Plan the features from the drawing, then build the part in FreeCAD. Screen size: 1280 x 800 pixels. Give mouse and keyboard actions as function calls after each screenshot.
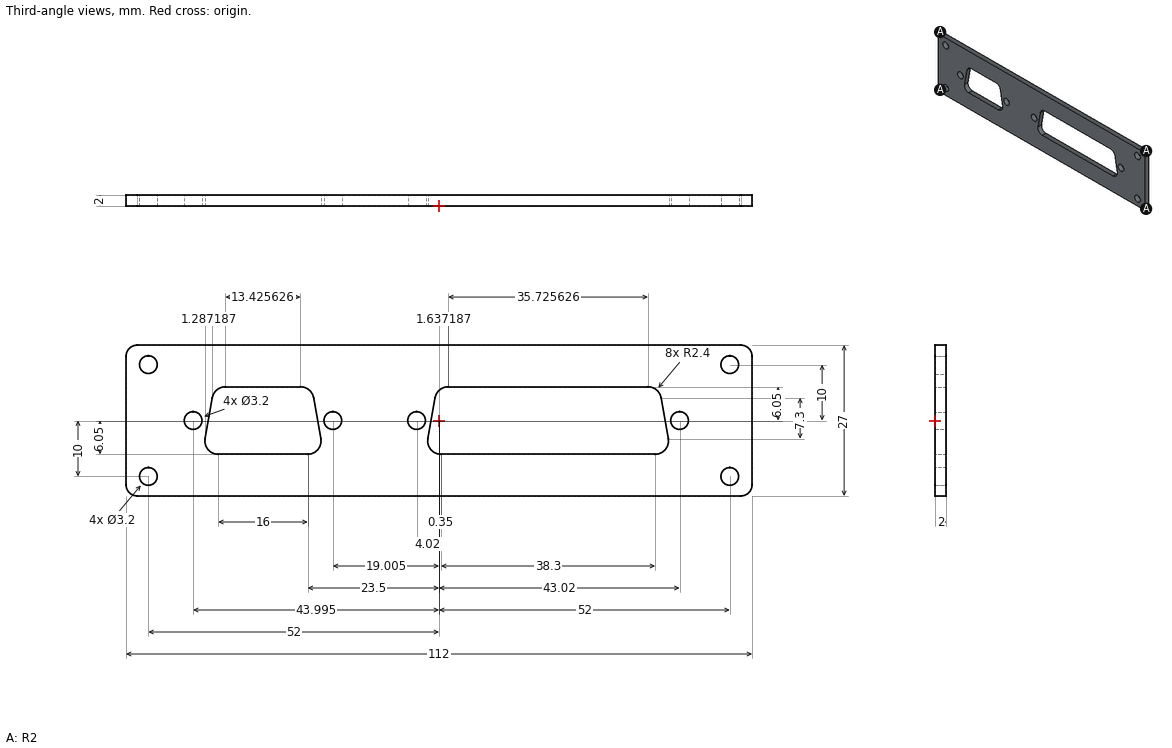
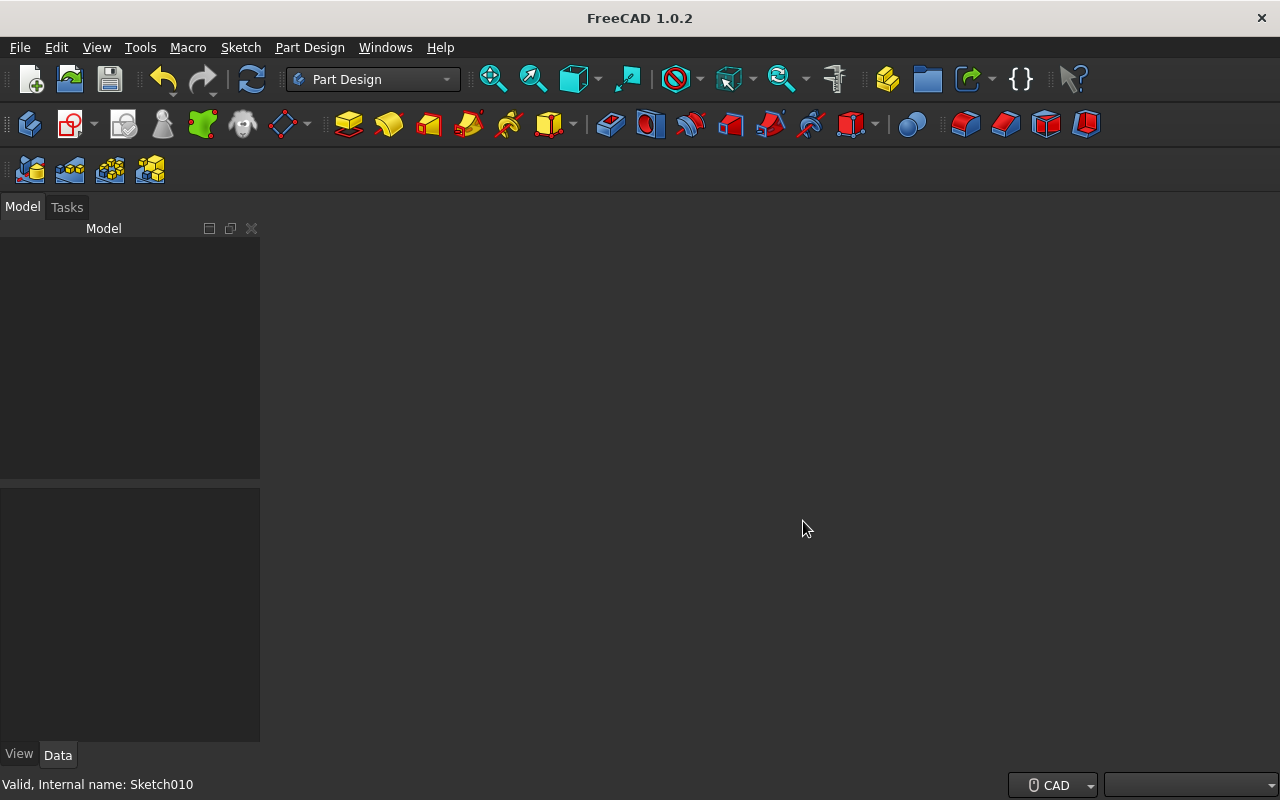
key(ctrl+n)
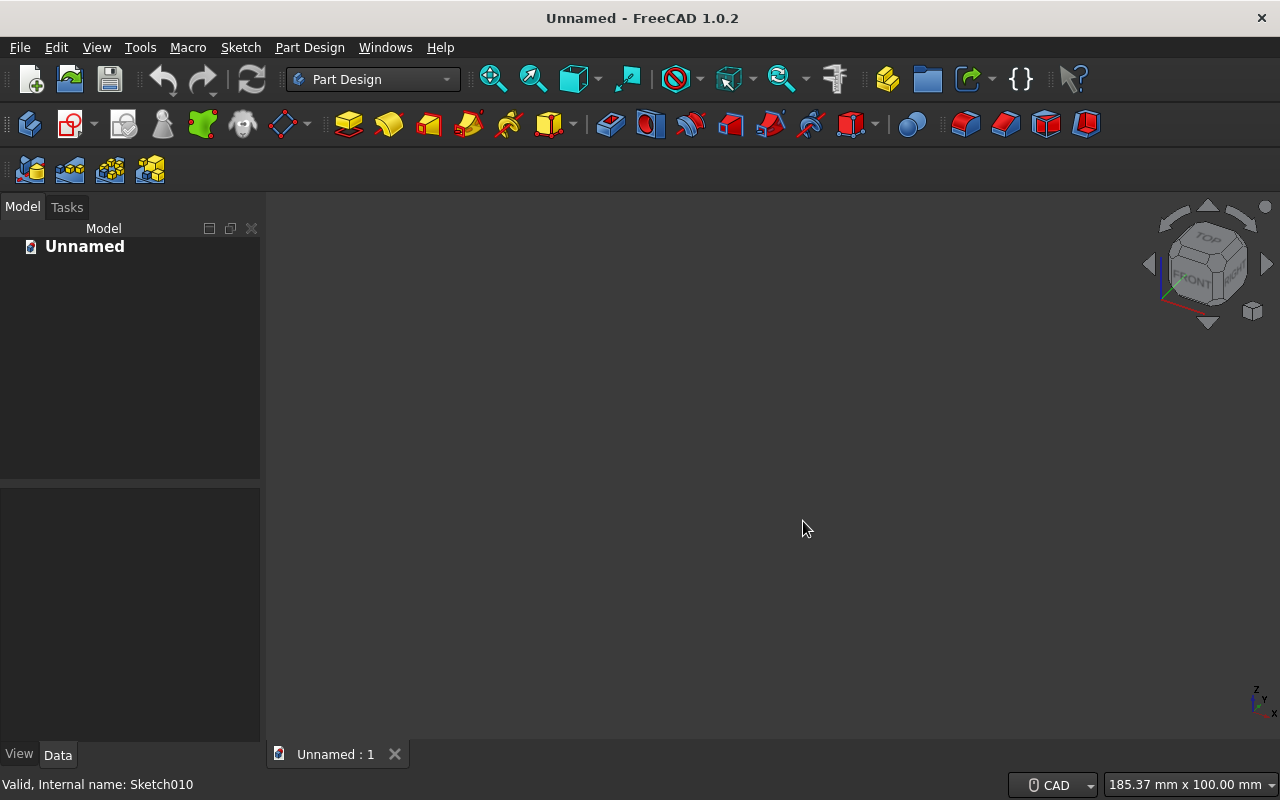
click(70, 124)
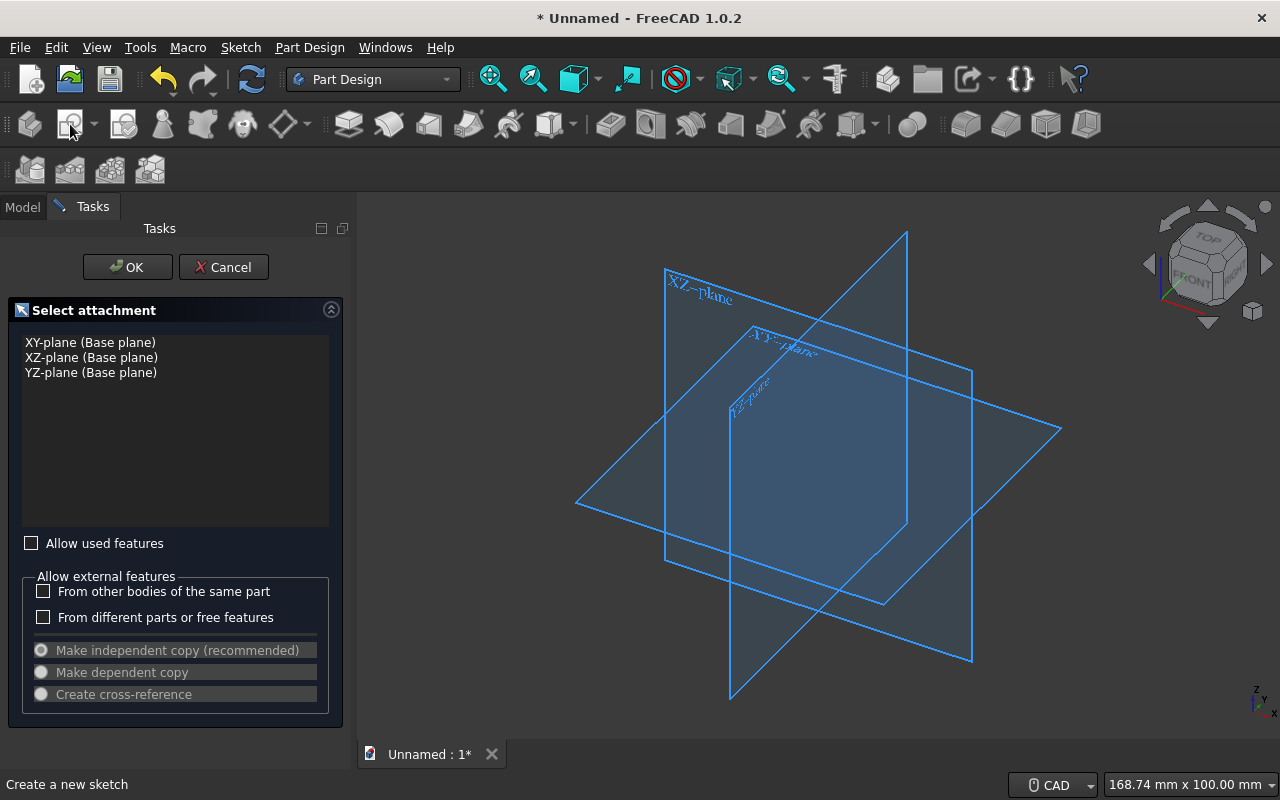
click(82, 358)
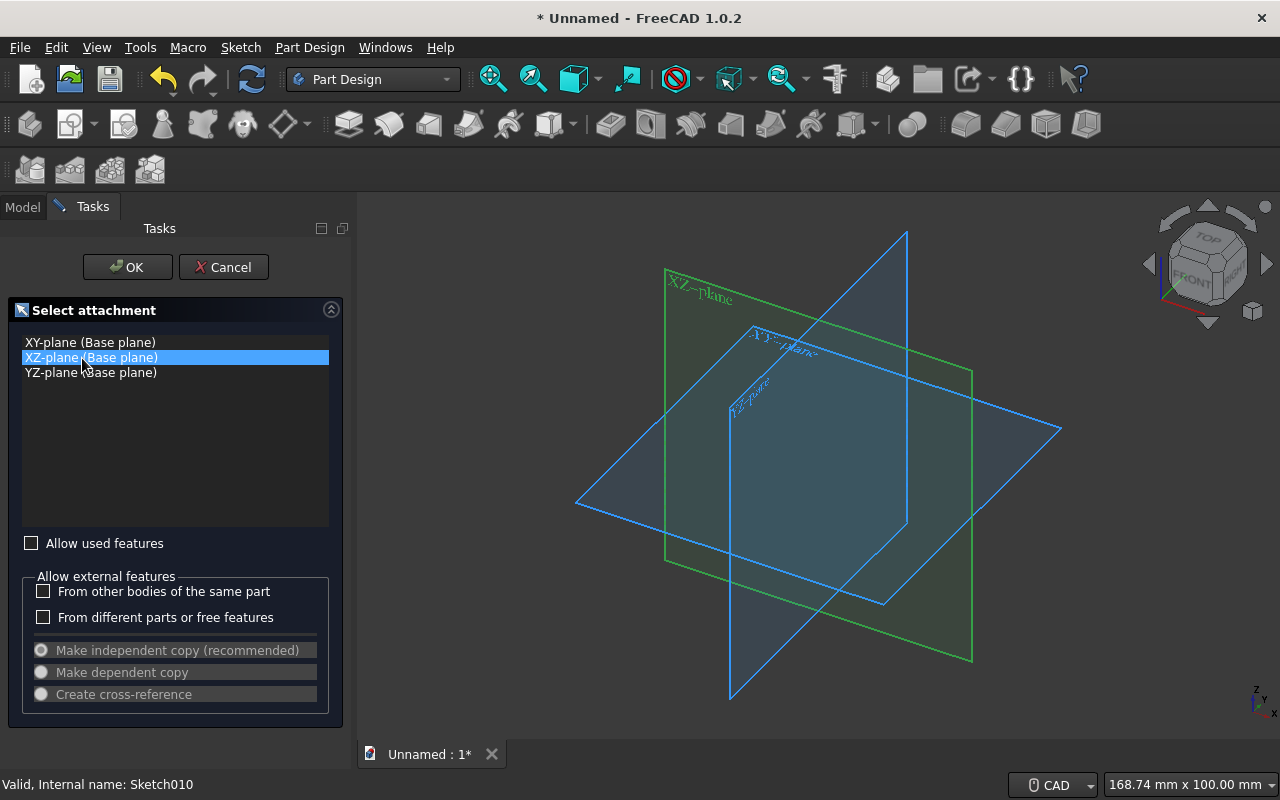
click(128, 267)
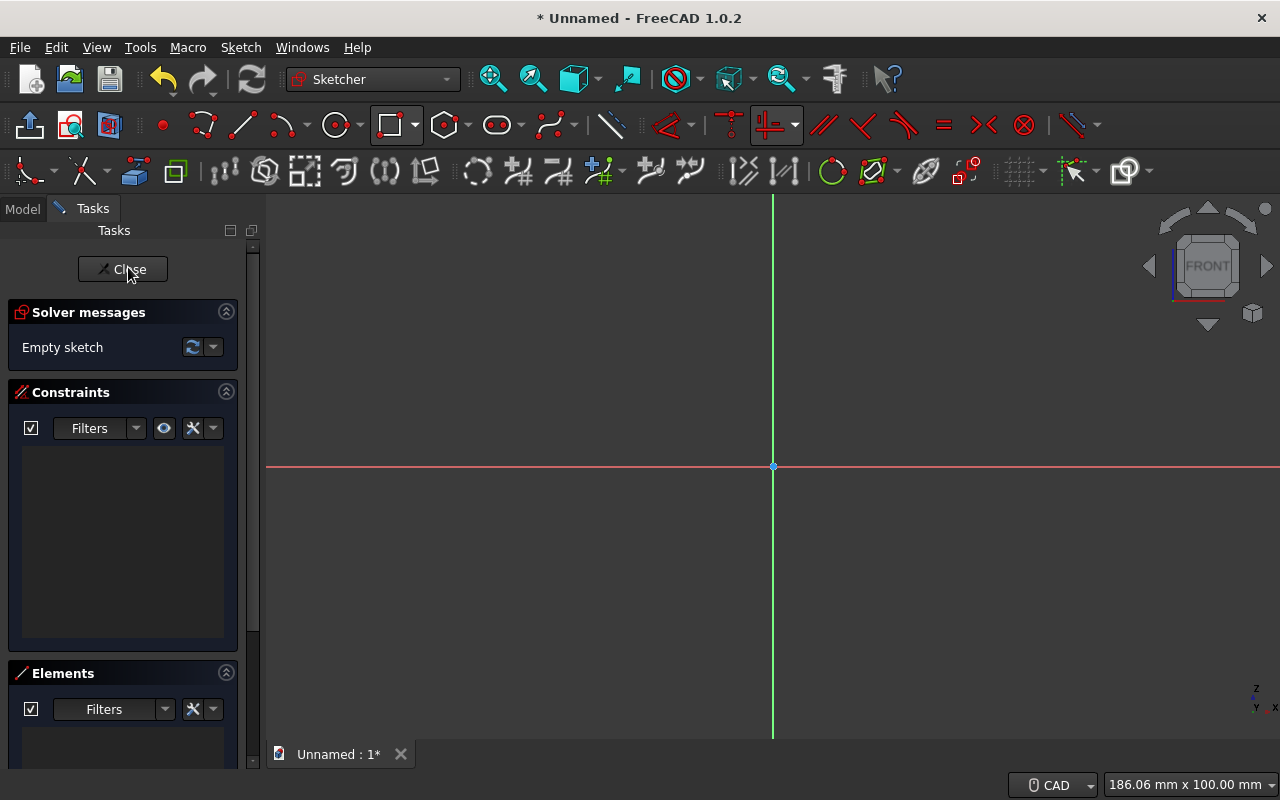
click(418, 126)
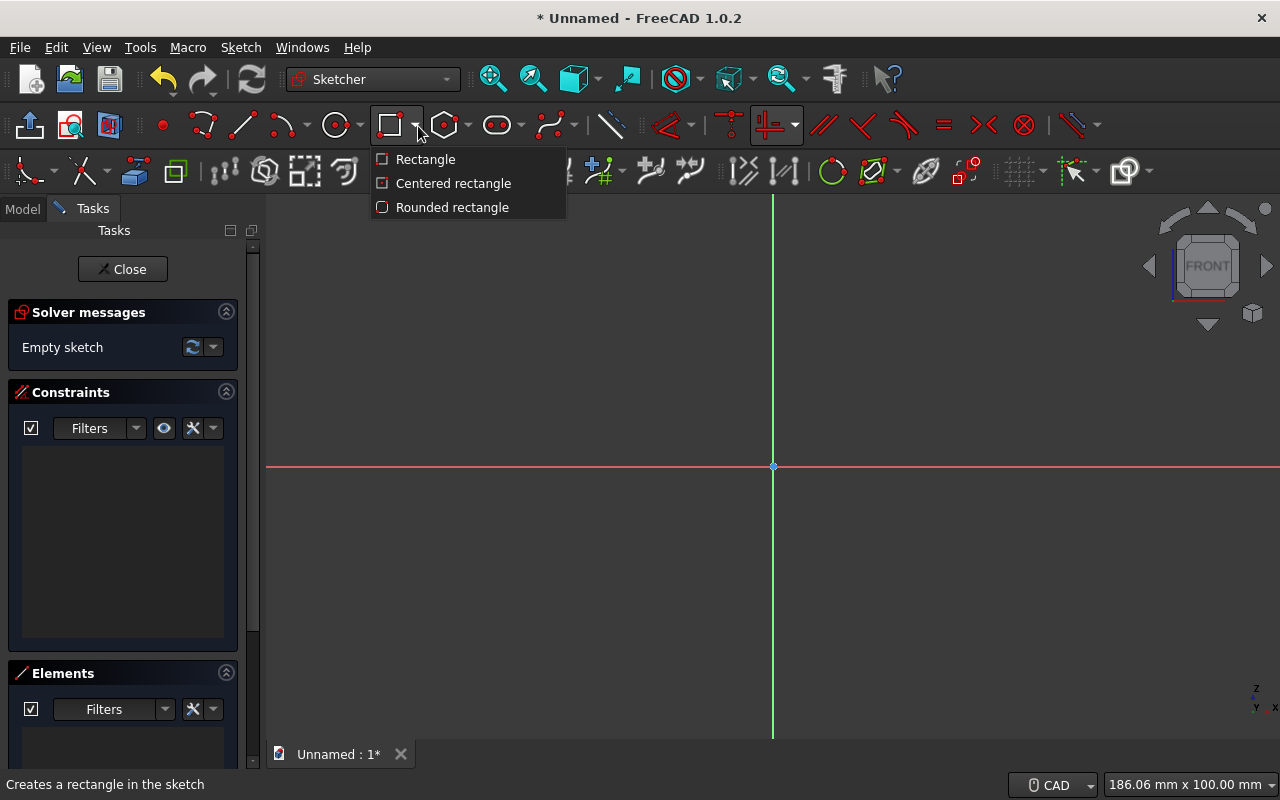
click(468, 183)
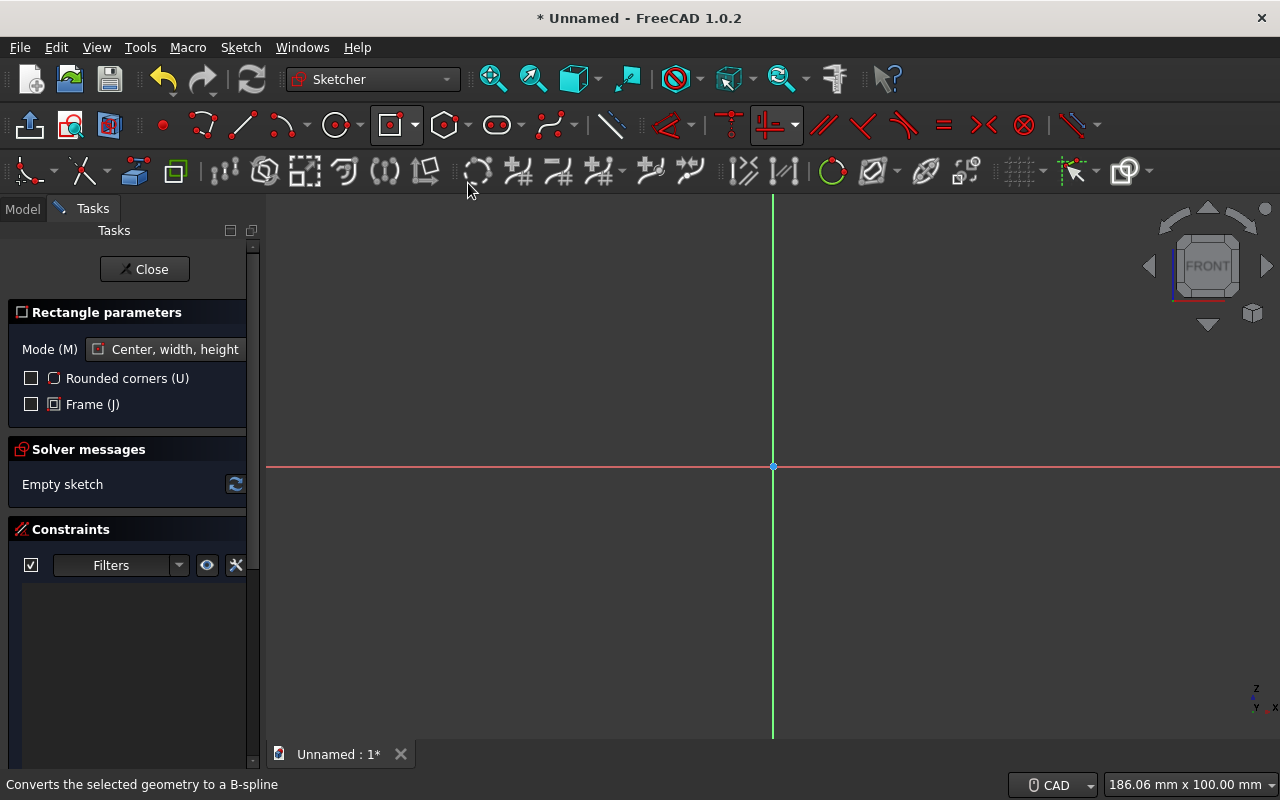
click(773, 466)
click(1078, 393)
key(Escape)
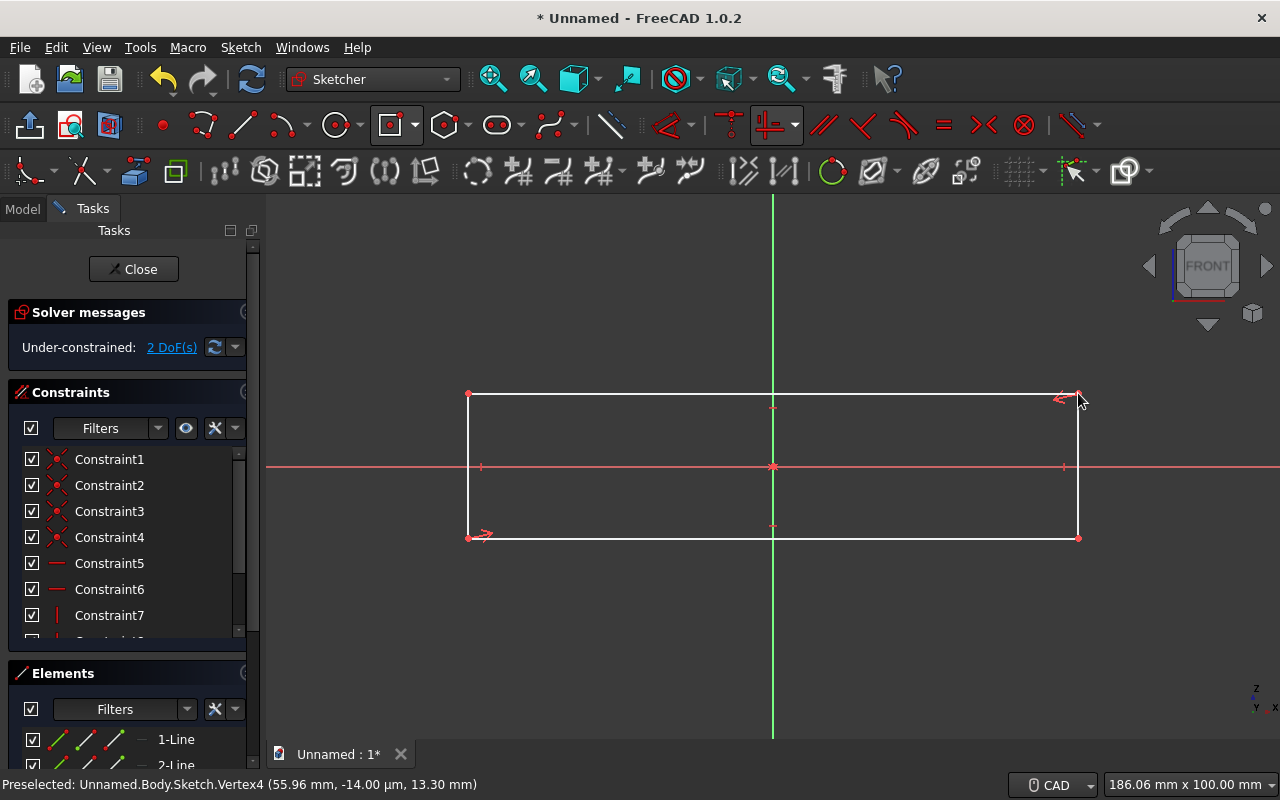
click(1078, 495)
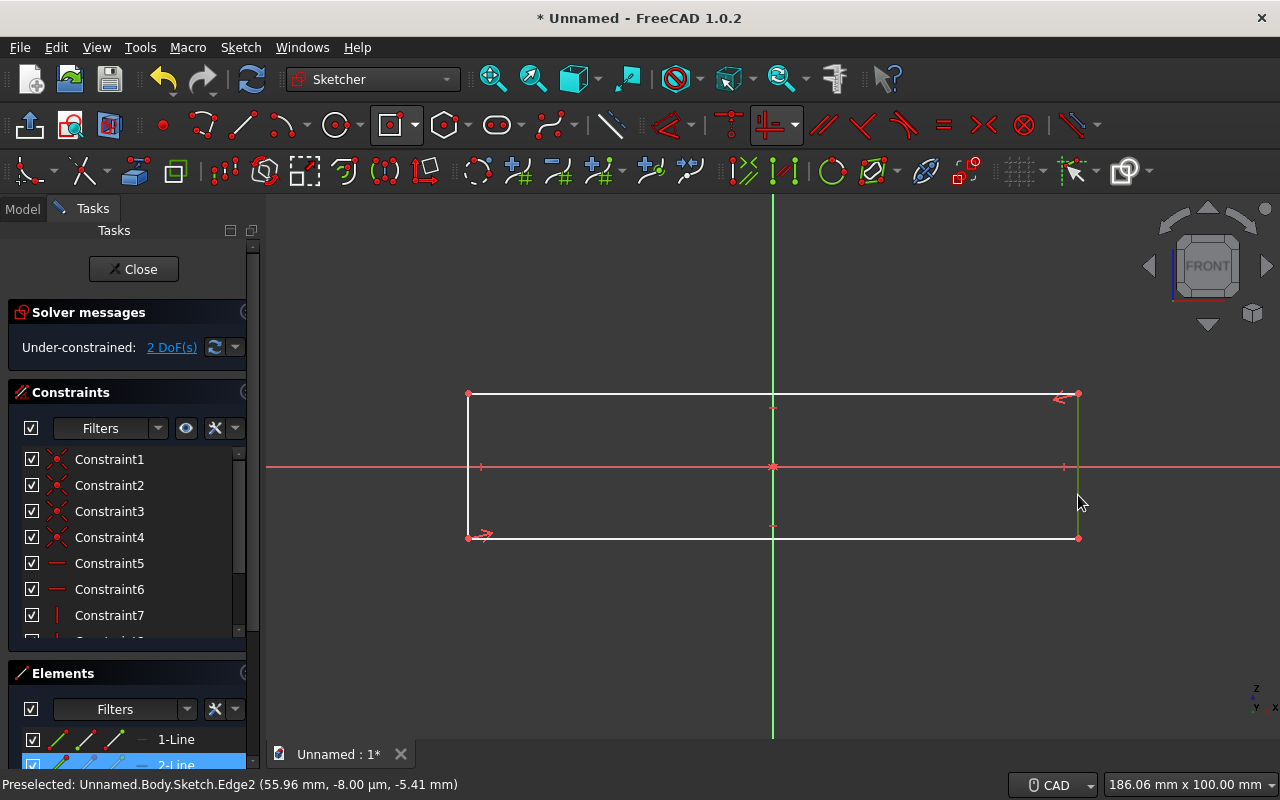
key(i)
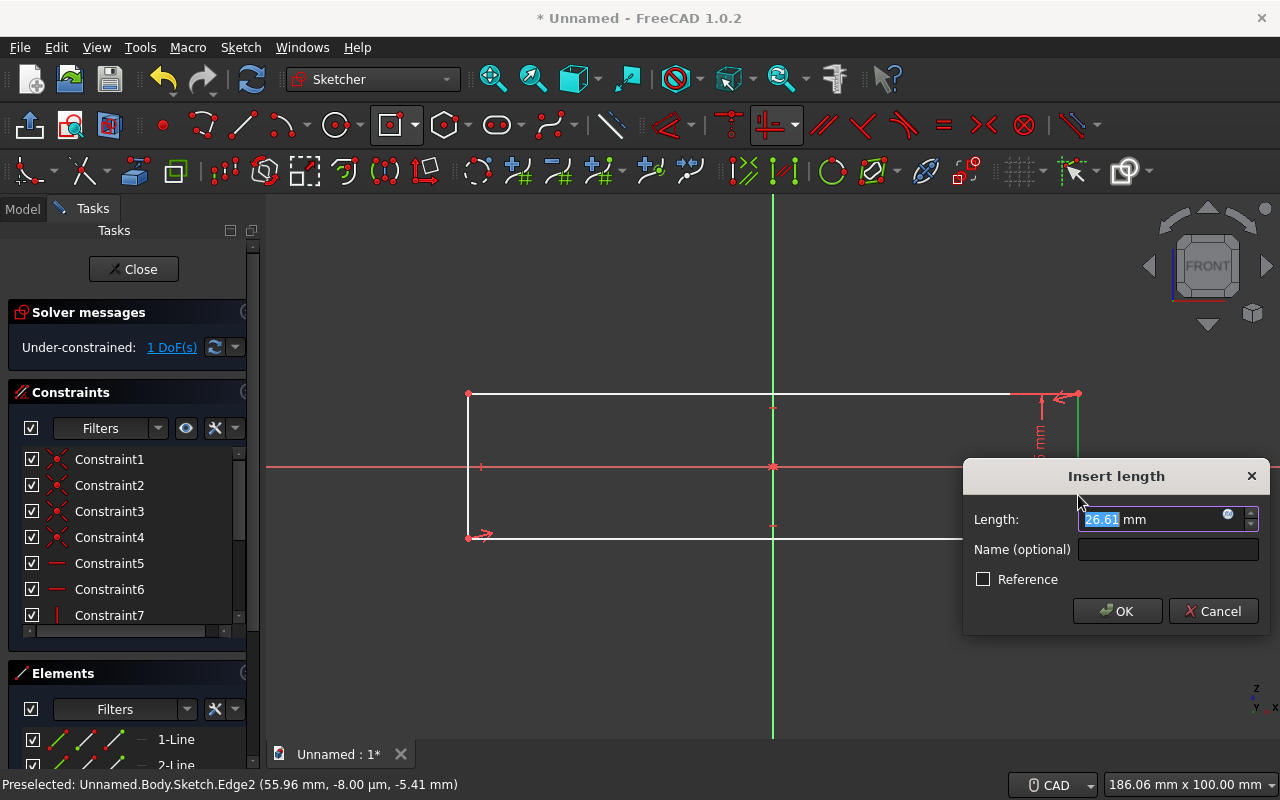
text(27)
key(Return)